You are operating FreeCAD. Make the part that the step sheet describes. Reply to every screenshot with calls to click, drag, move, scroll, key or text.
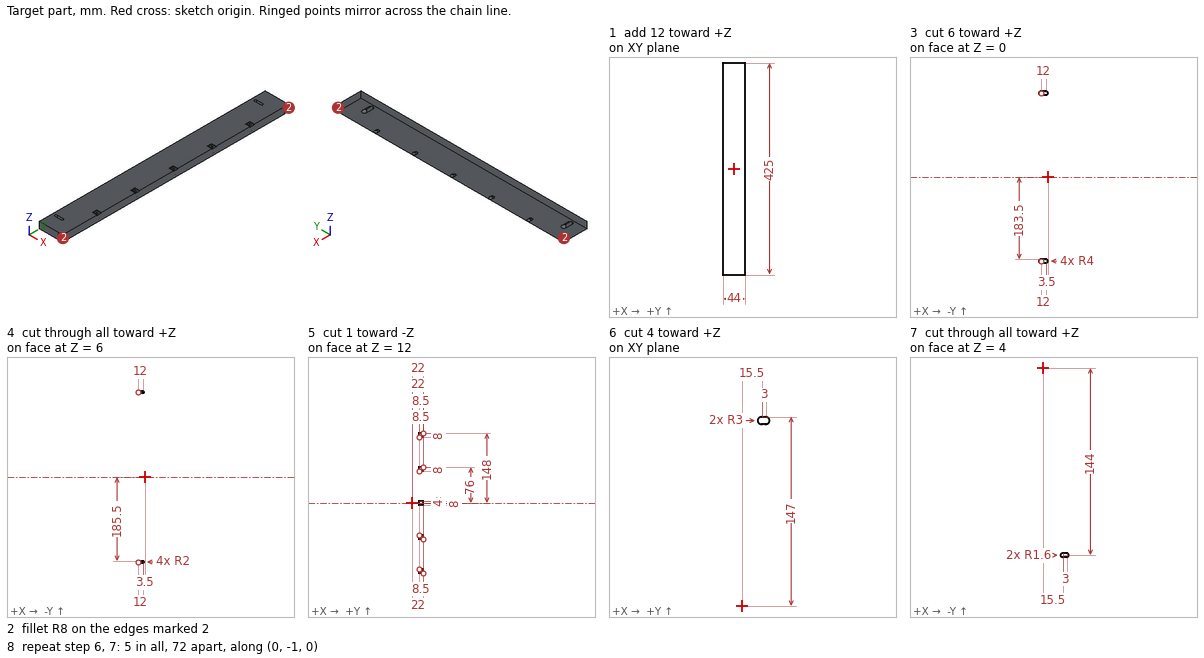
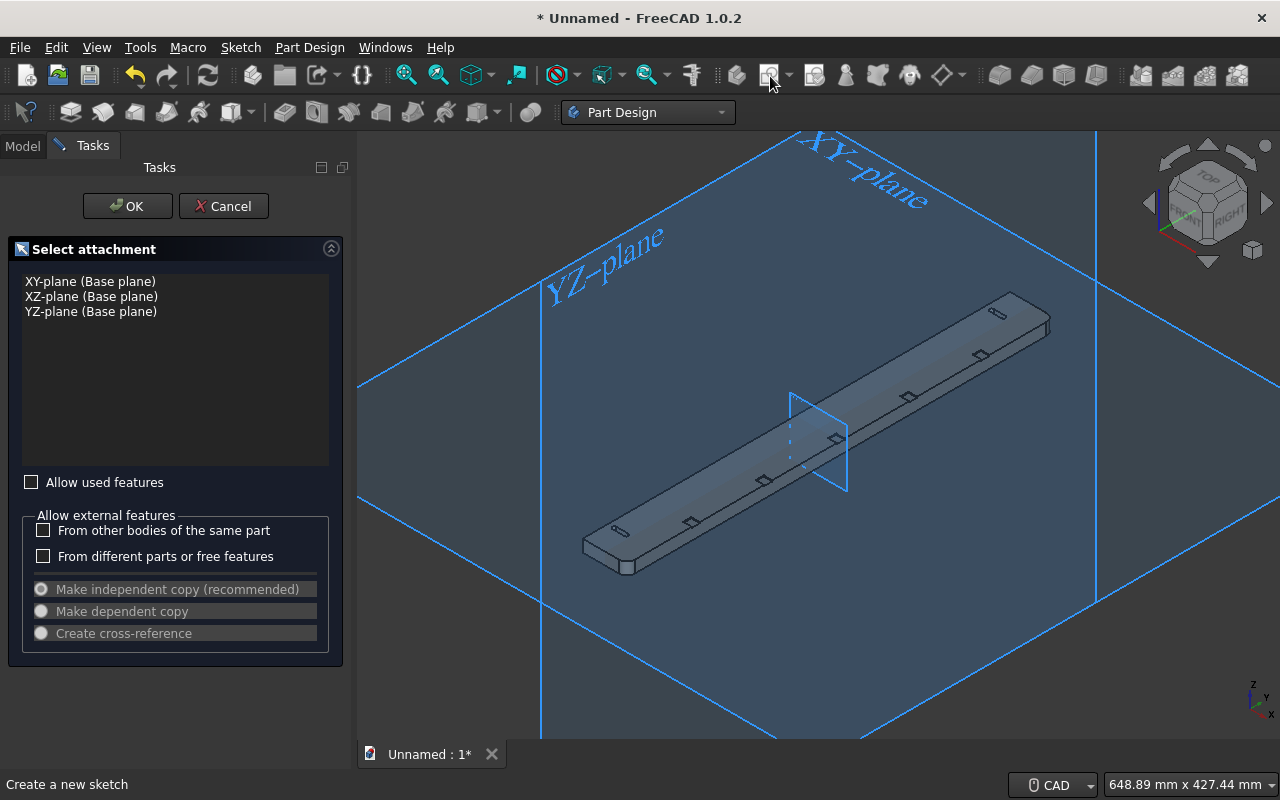
click(82, 282)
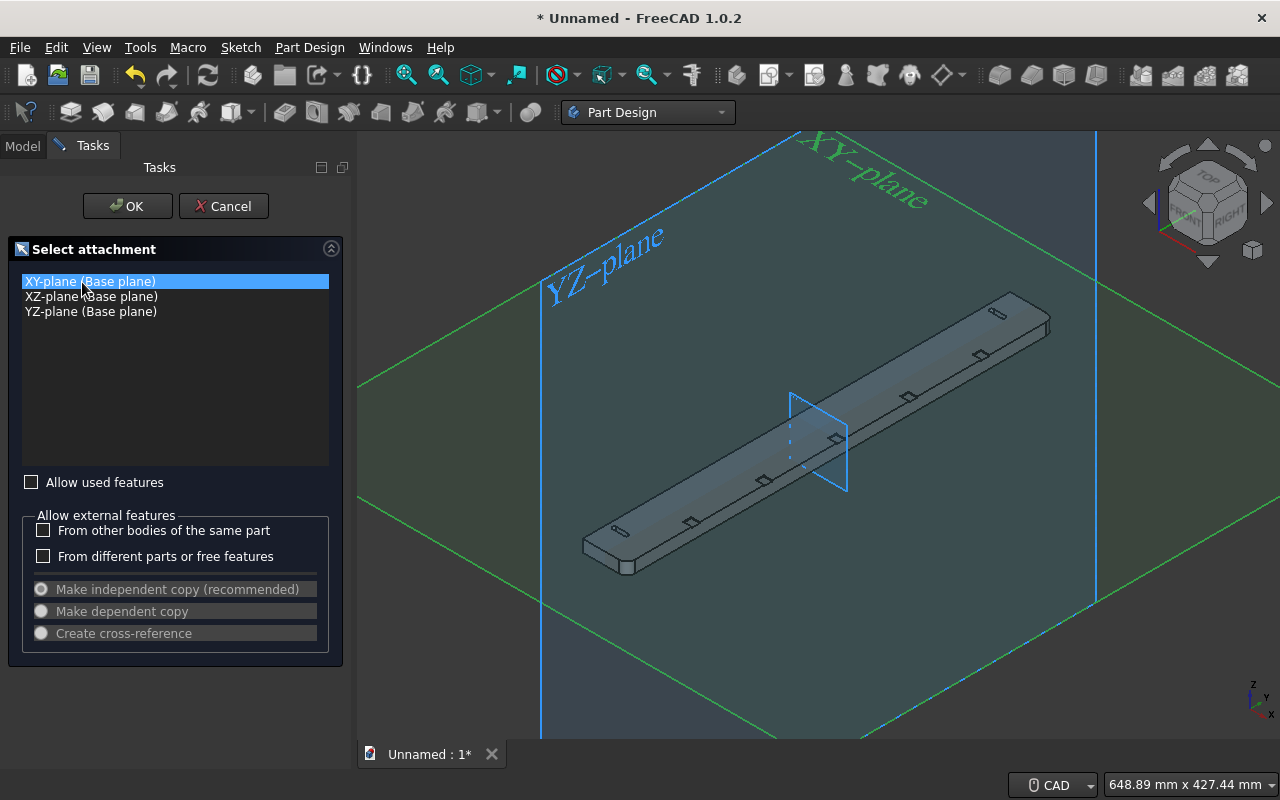
click(128, 206)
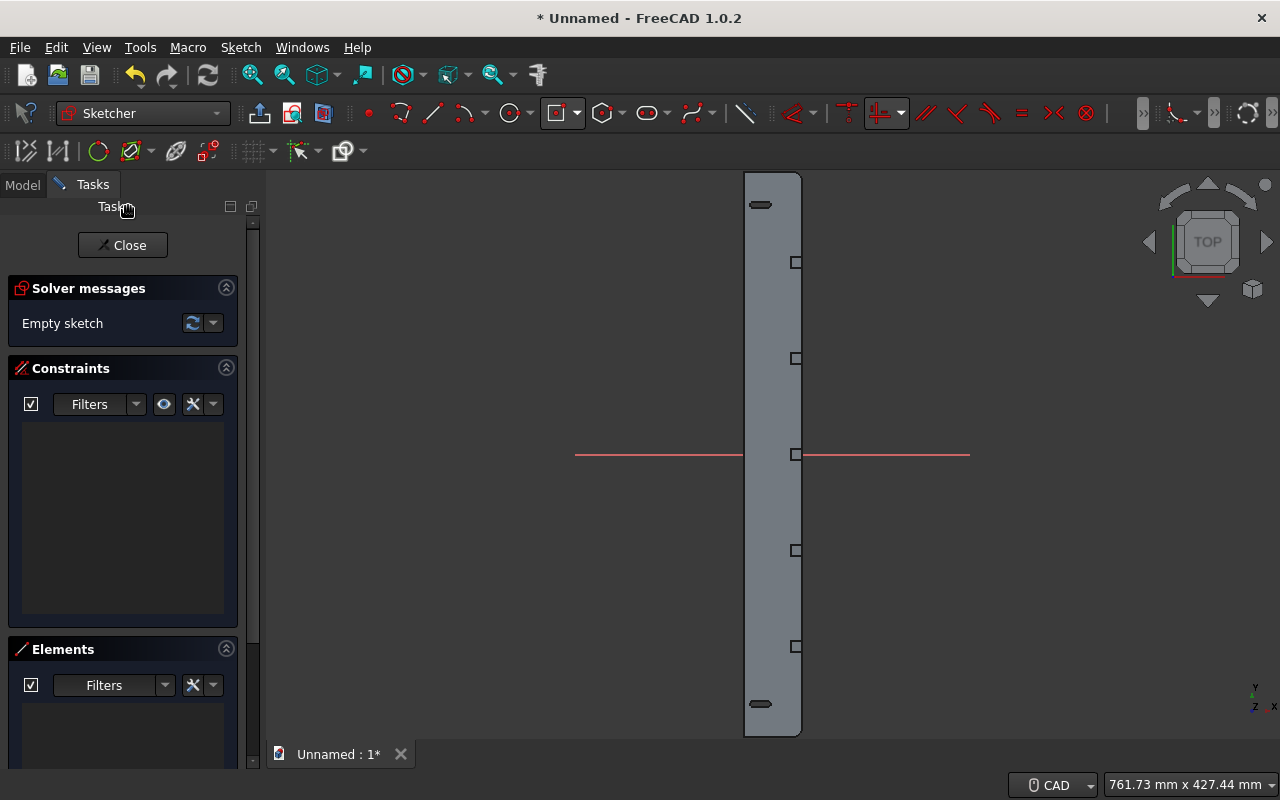
click(324, 114)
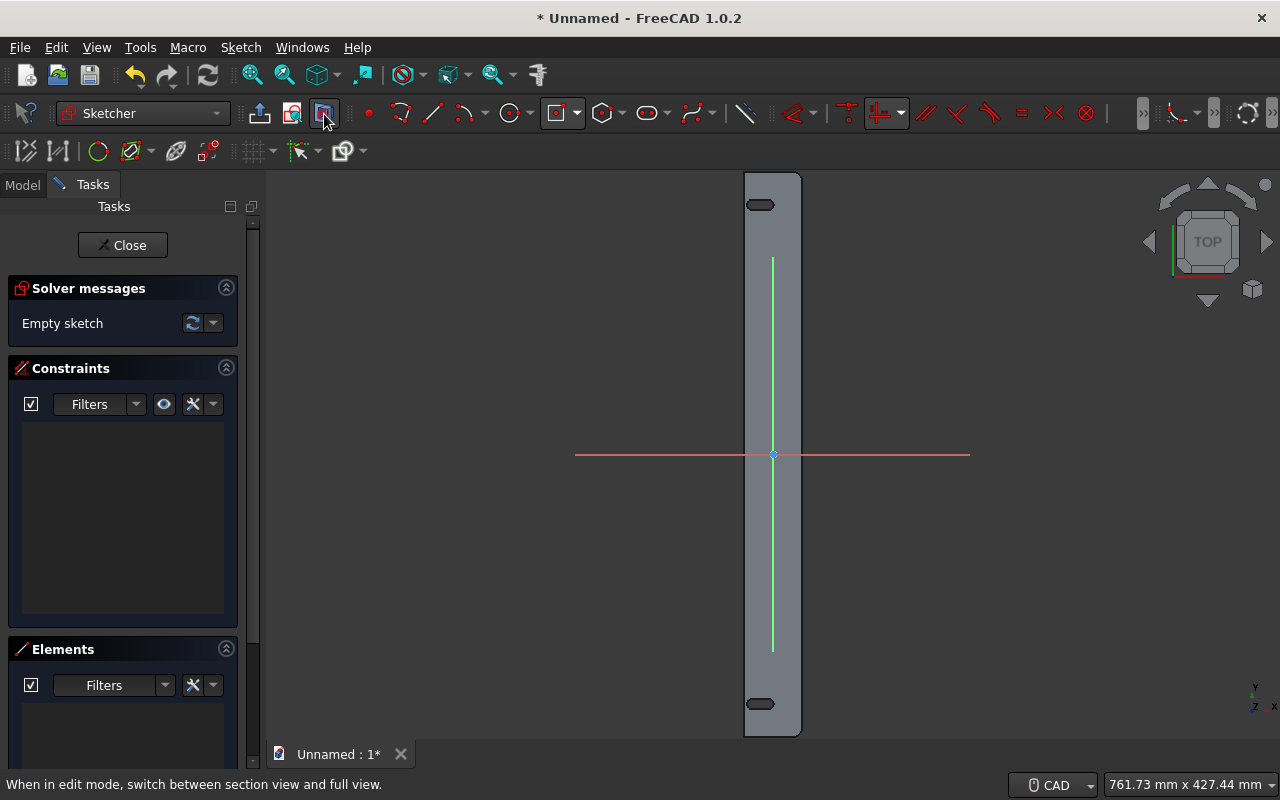
scroll(800, 253, up, 15)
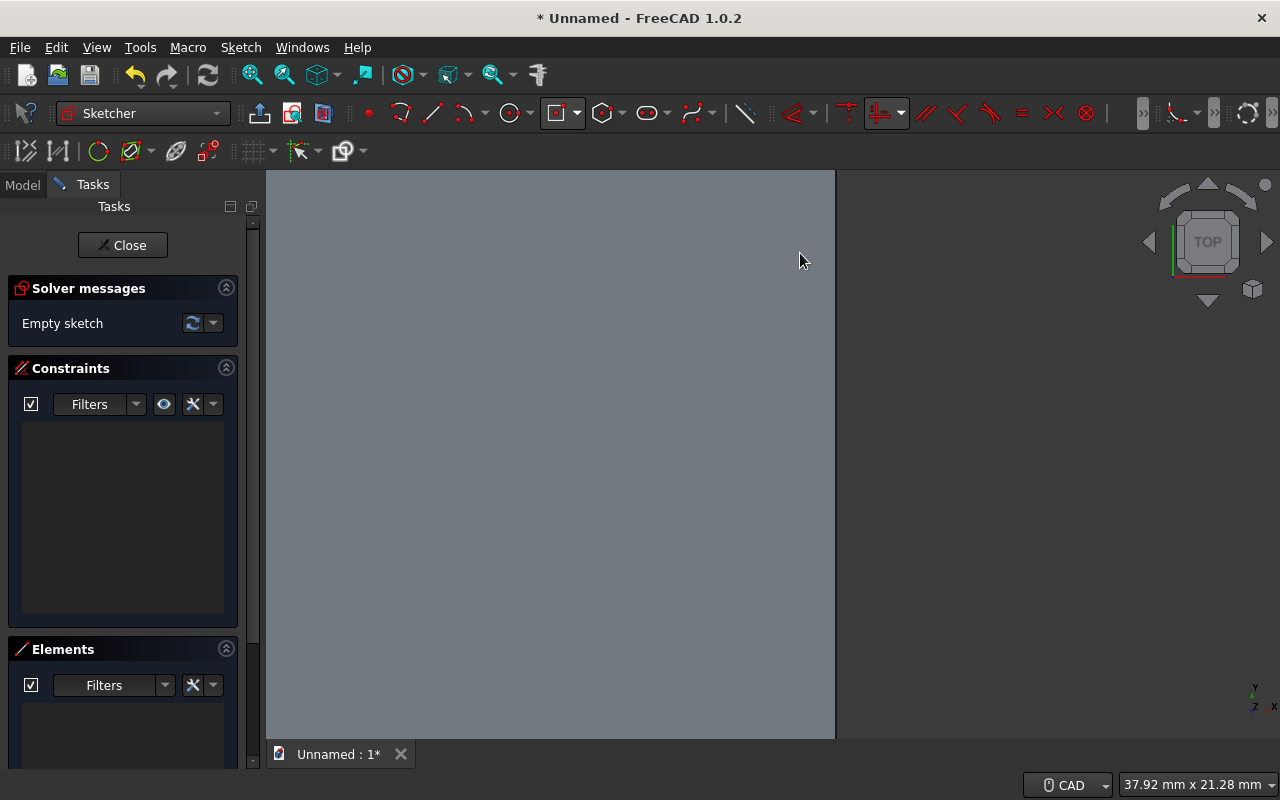
scroll(700, 441, up, 4)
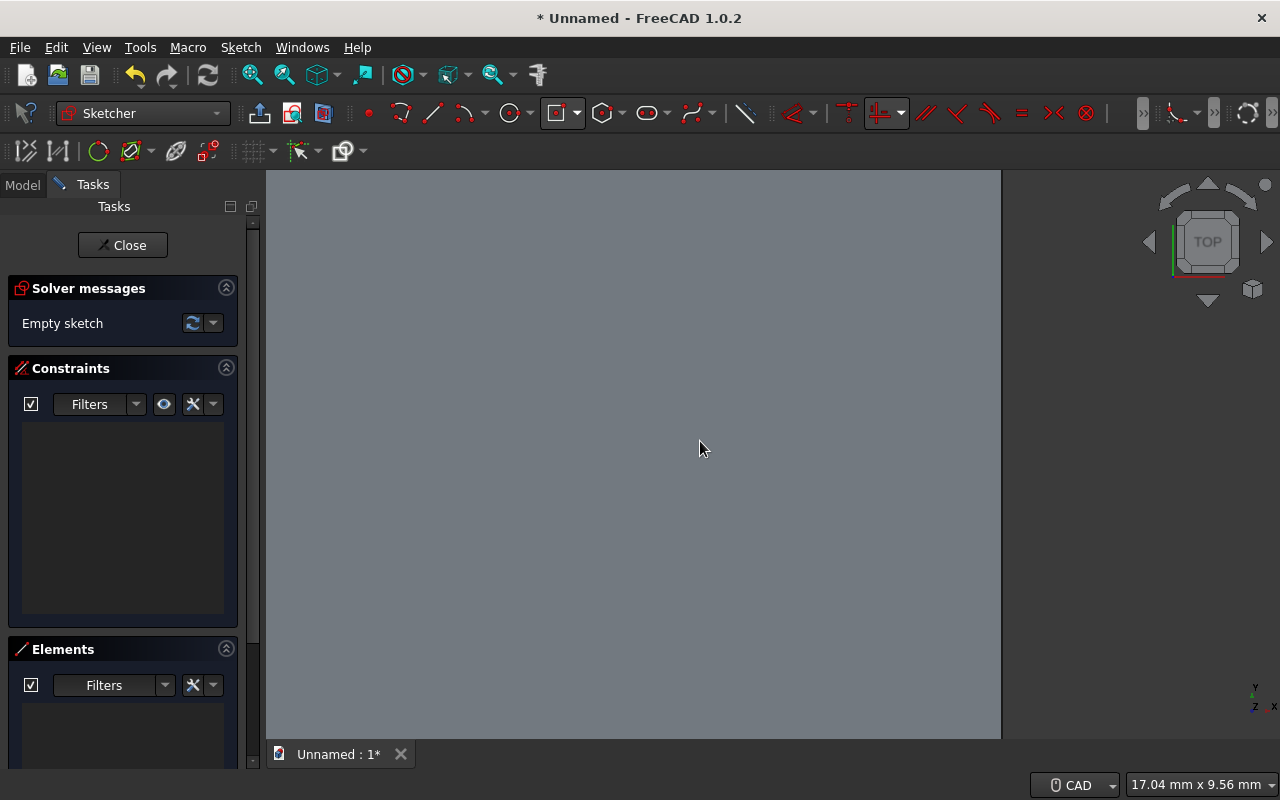
key(g)
key(s)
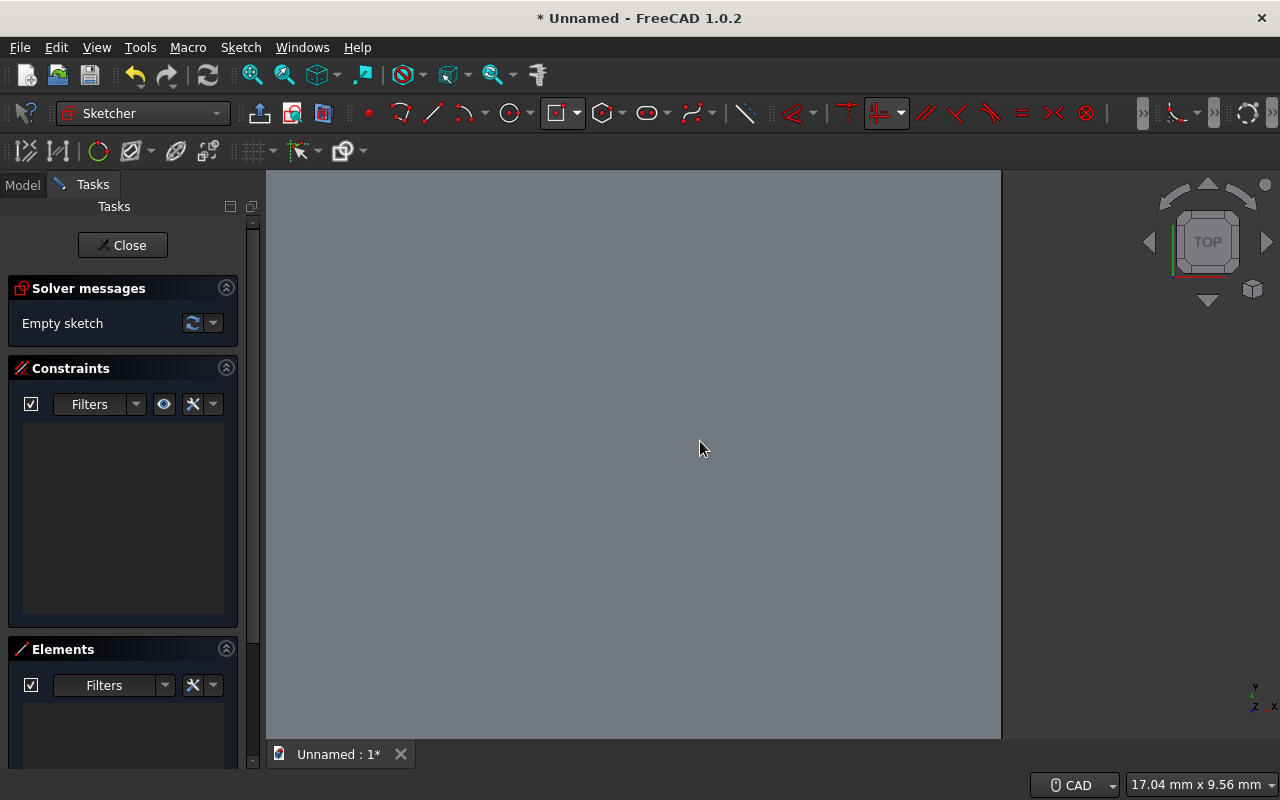
click(615, 454)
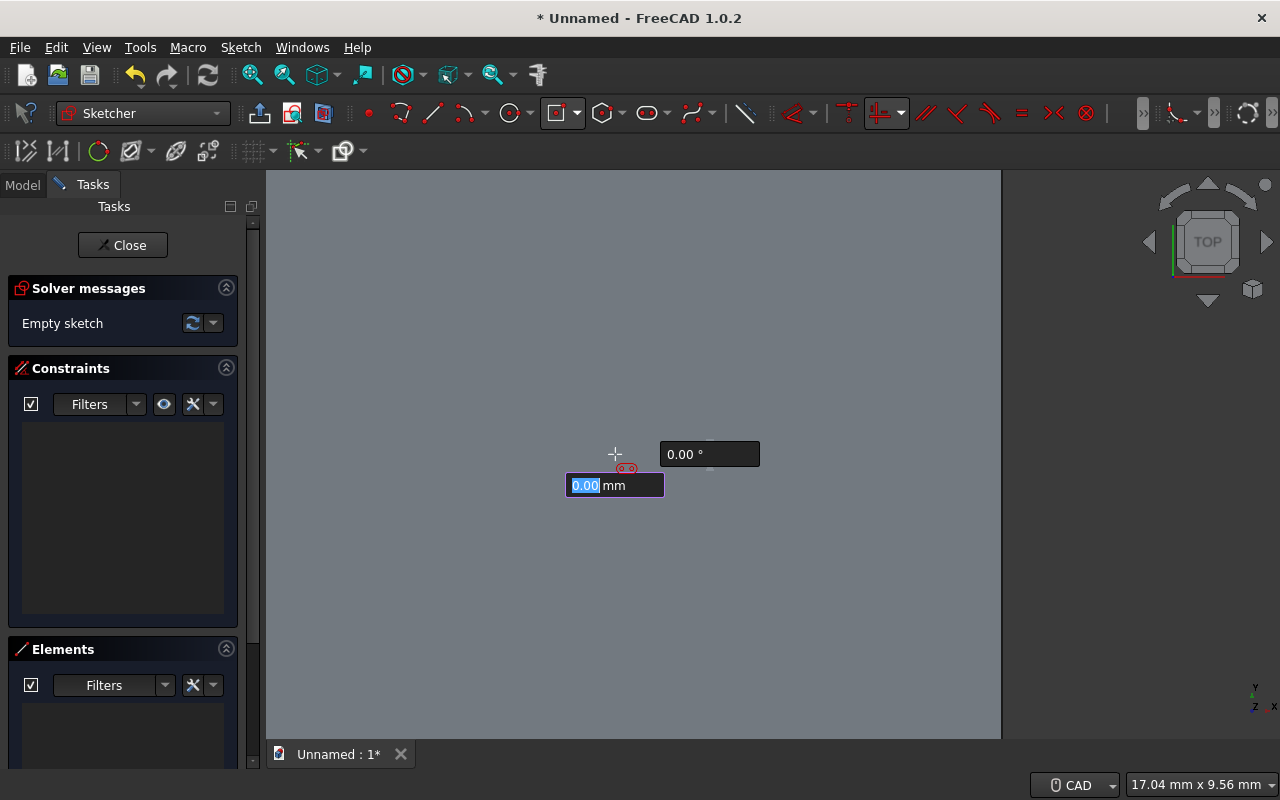
click(794, 454)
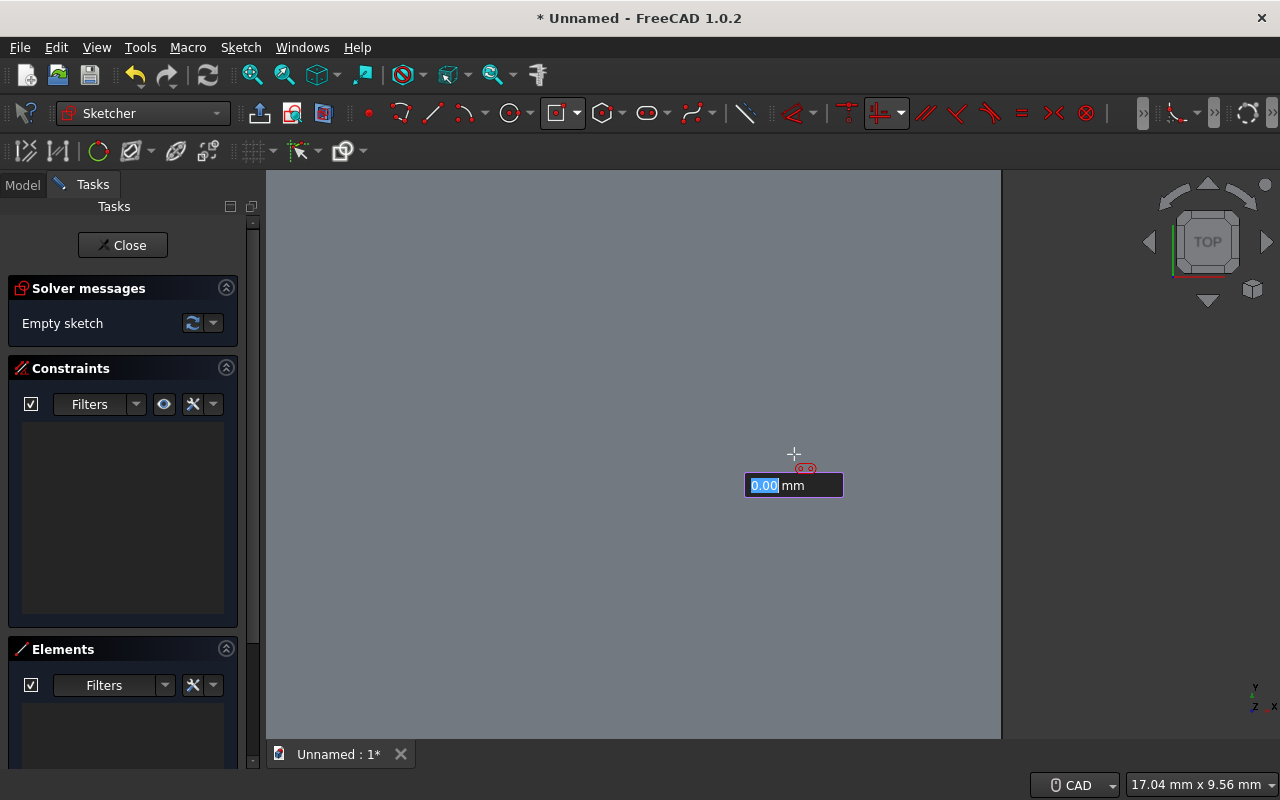
click(704, 276)
key(Escape)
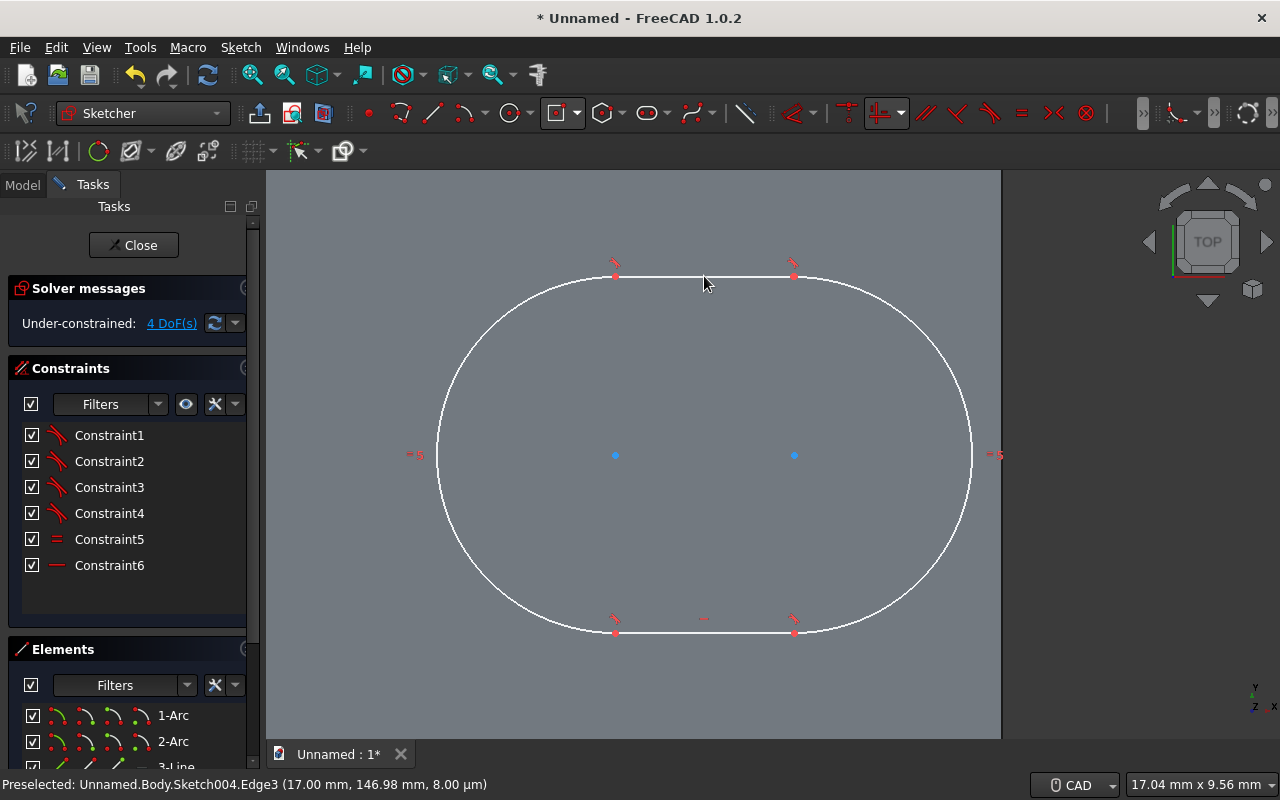
click(792, 114)